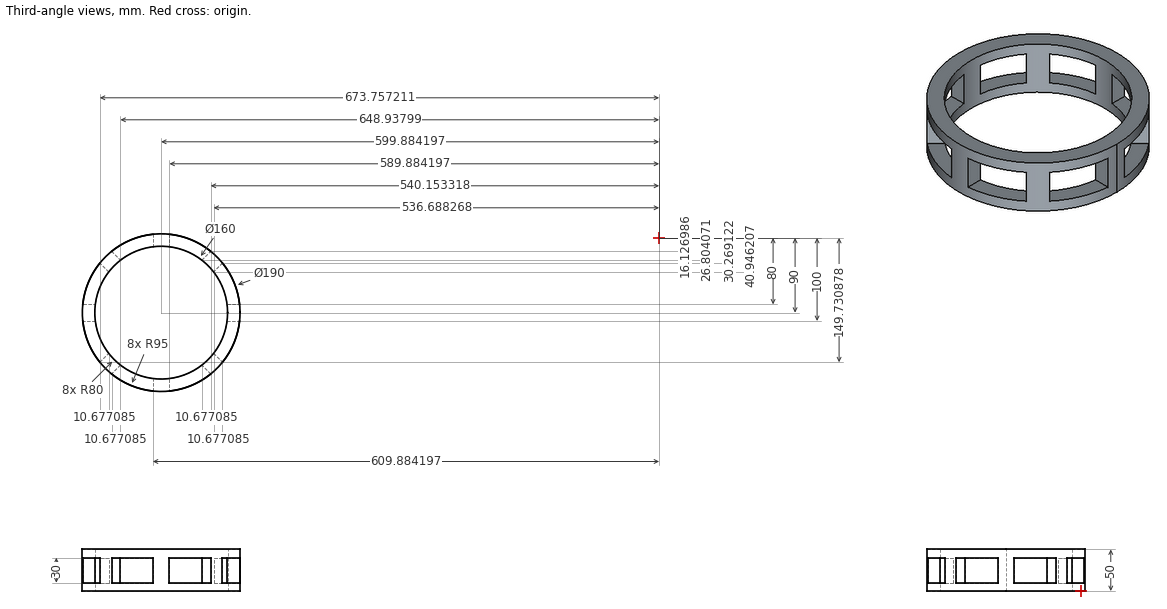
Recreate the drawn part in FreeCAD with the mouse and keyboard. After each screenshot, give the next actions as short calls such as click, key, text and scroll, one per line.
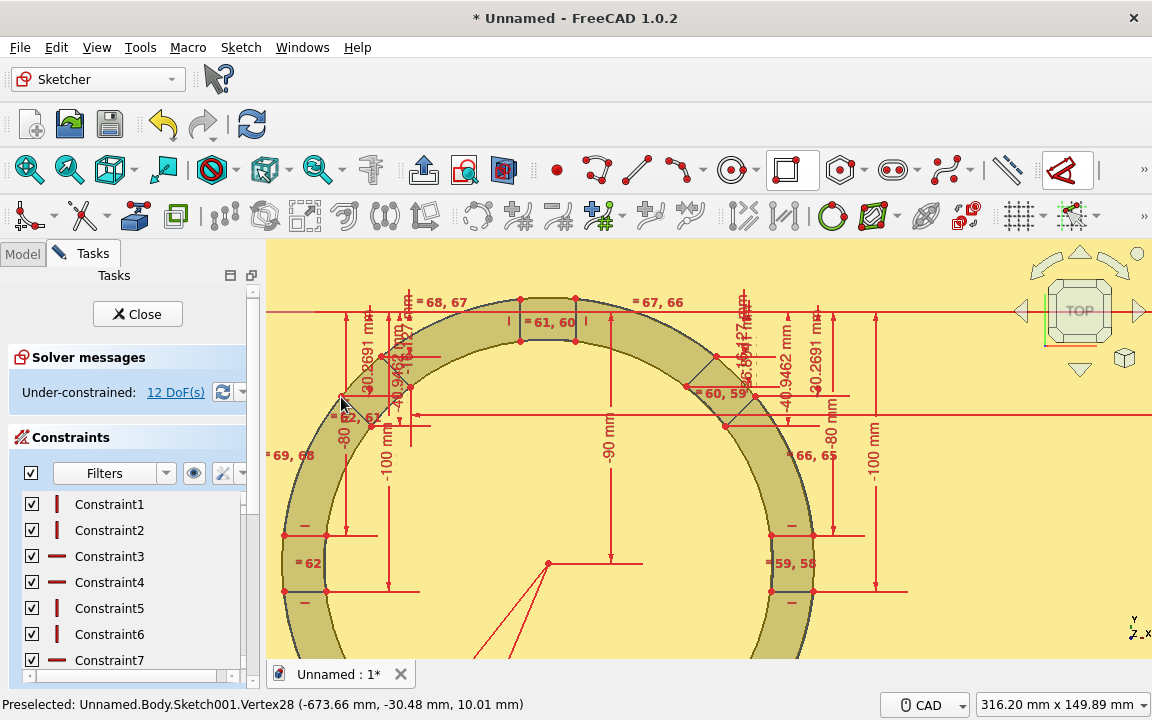
scroll(716, 355, down, 4)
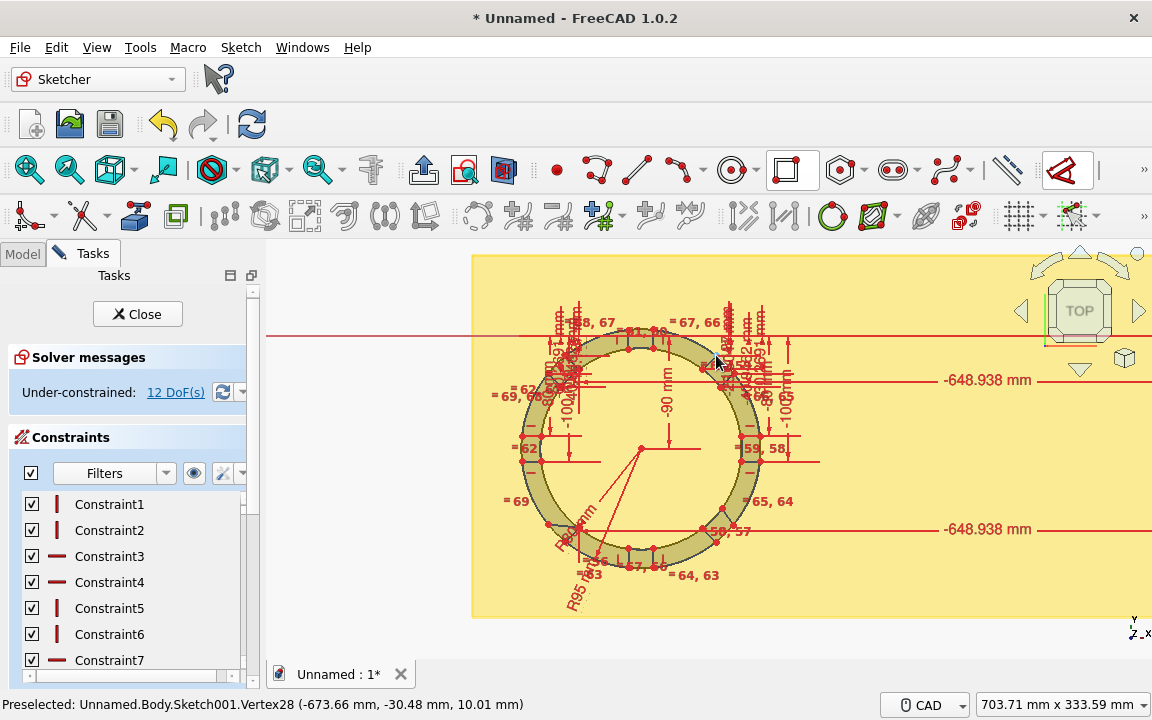
scroll(557, 525, up, 6)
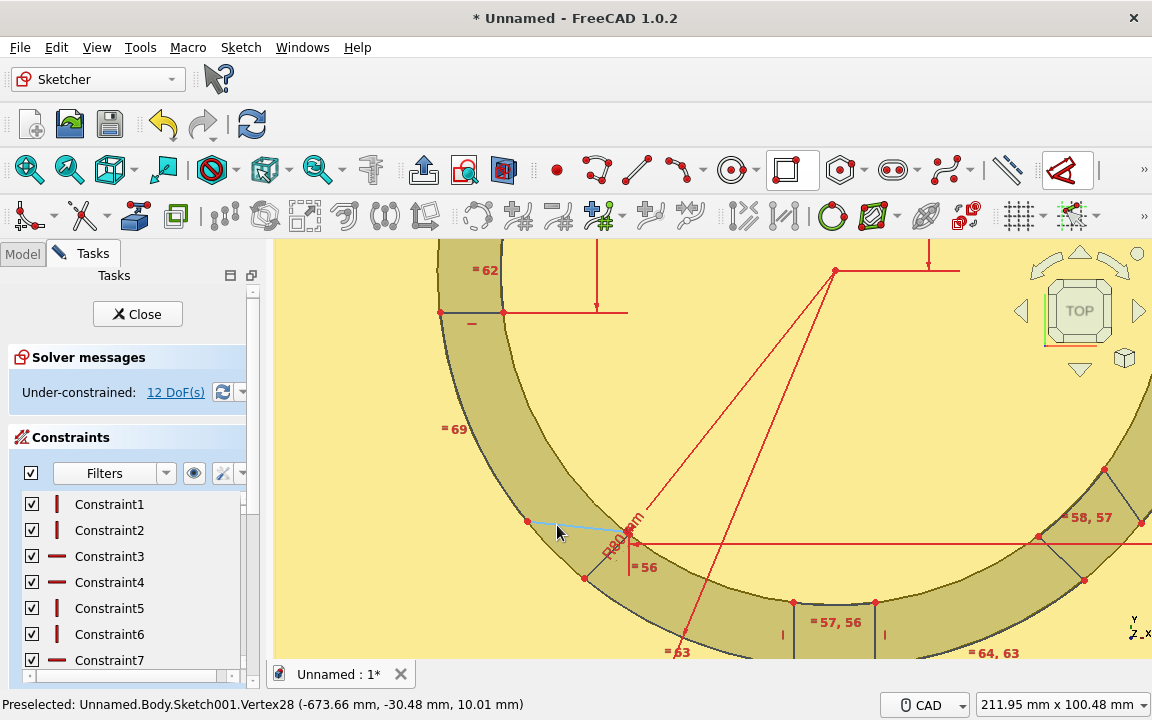
click(557, 525)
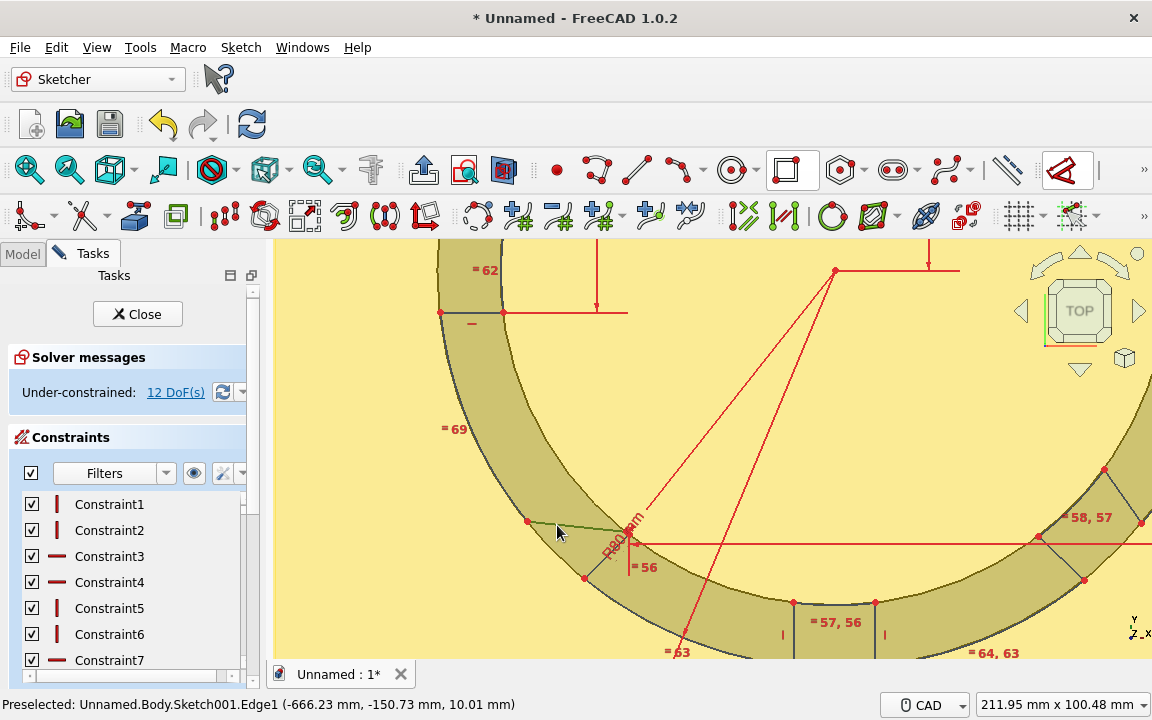
key(l)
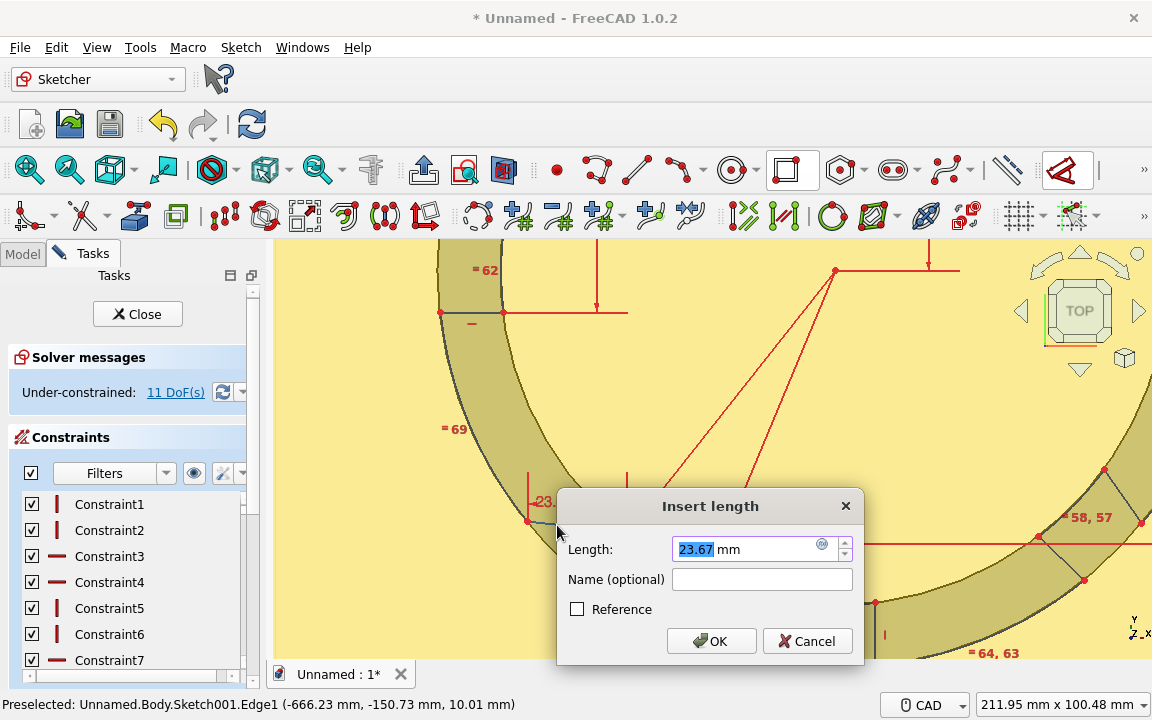
text(10.677085)
key(Return)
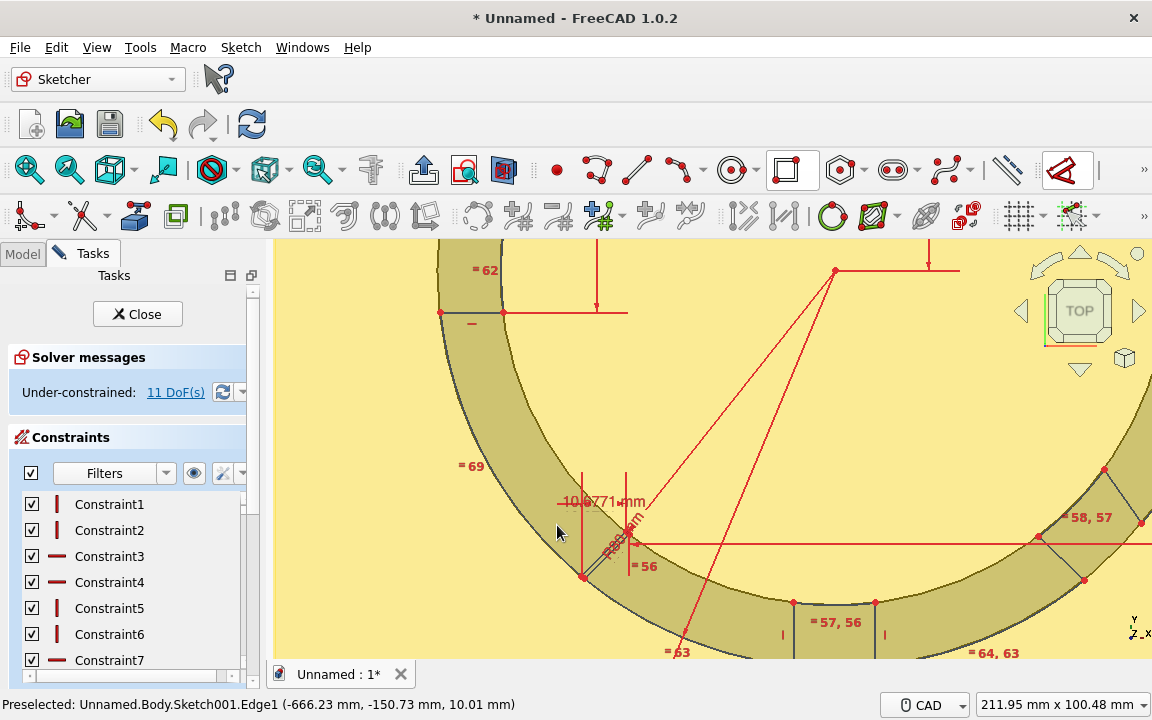
scroll(620, 543, up, 7)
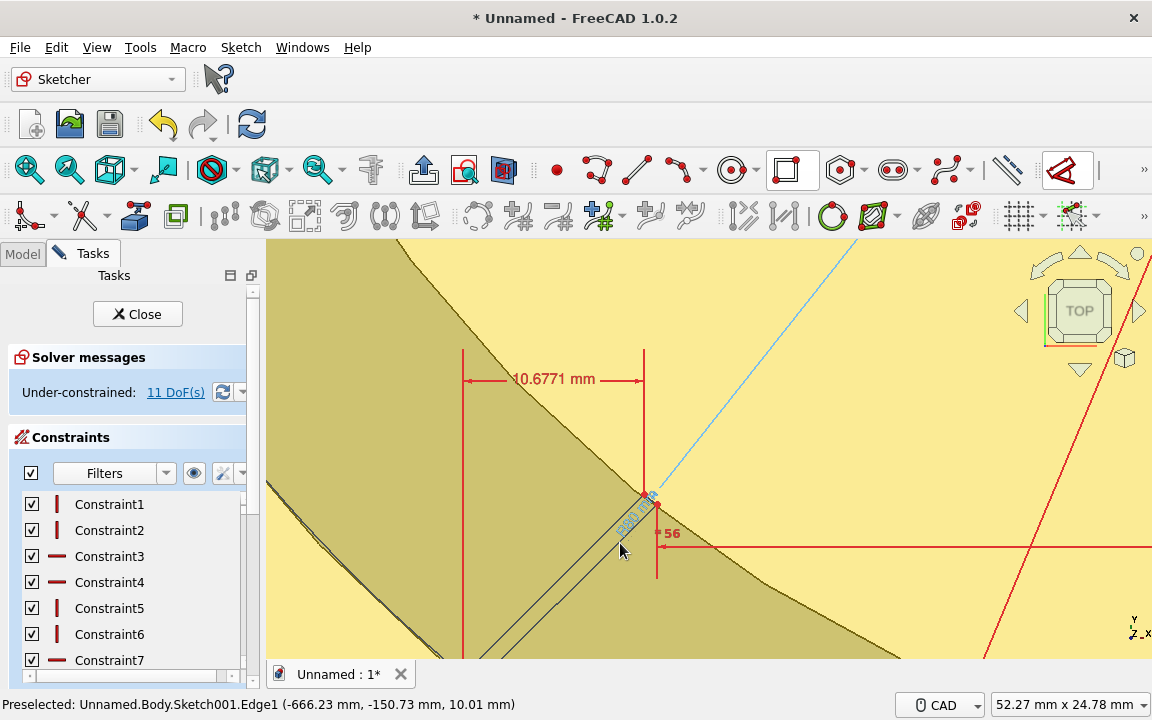
click(621, 541)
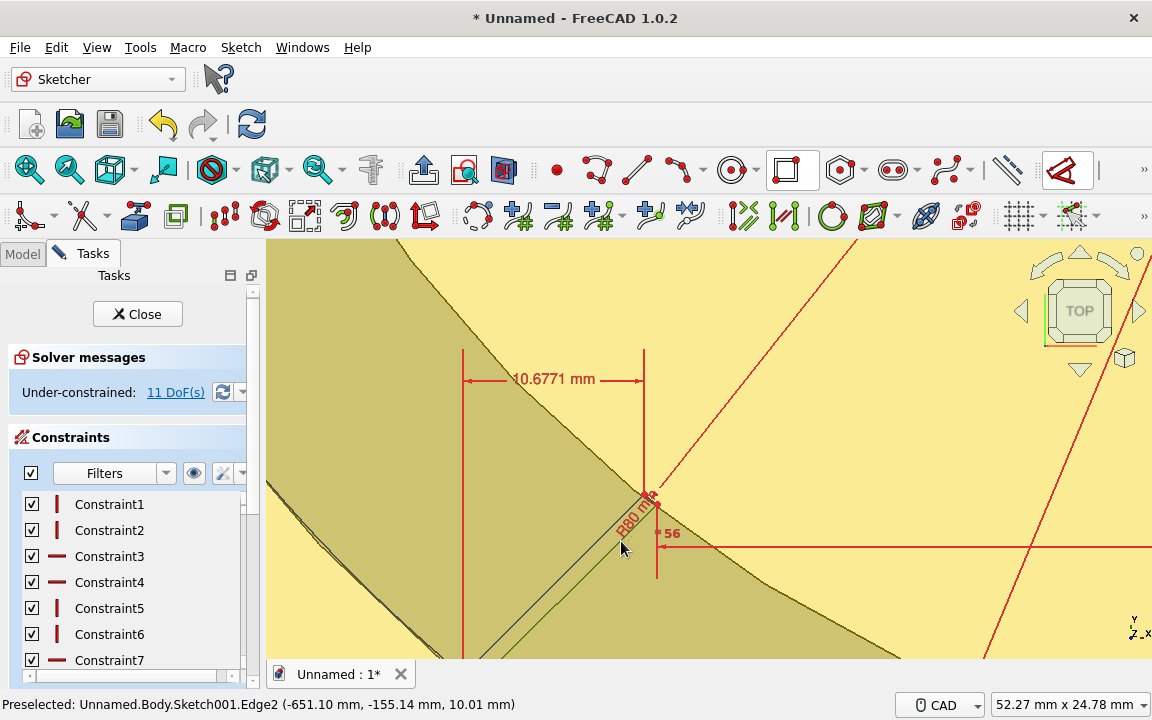
key(l)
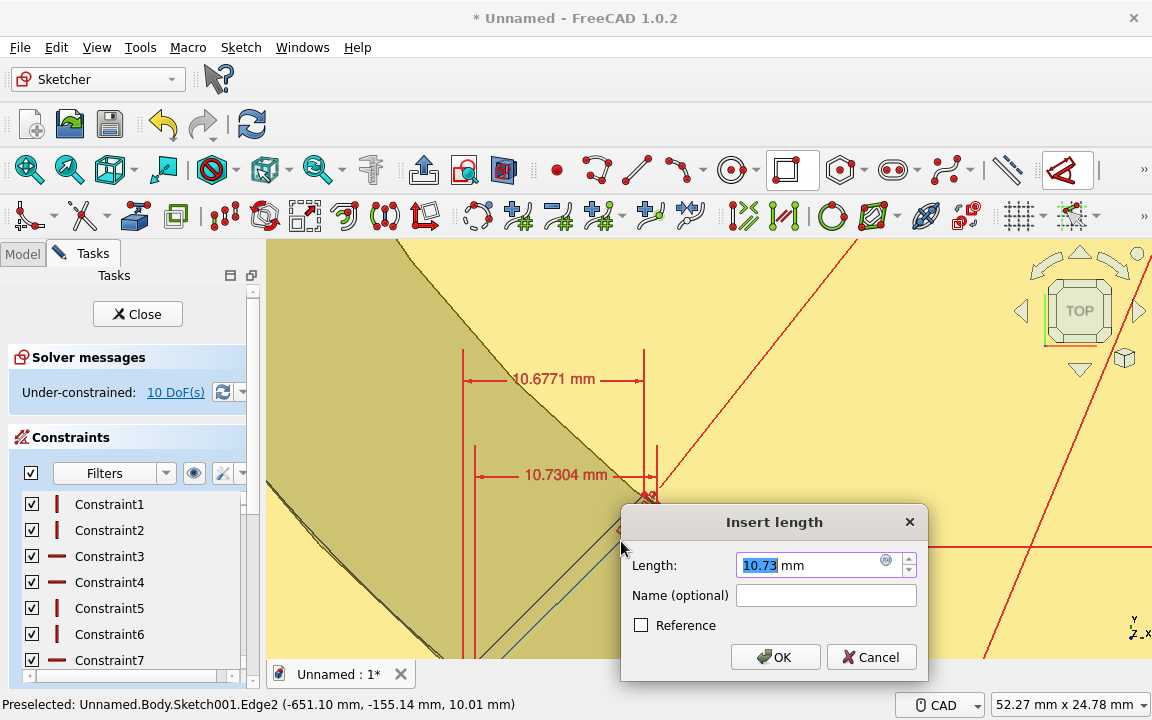
text(10.677085)
key(Return)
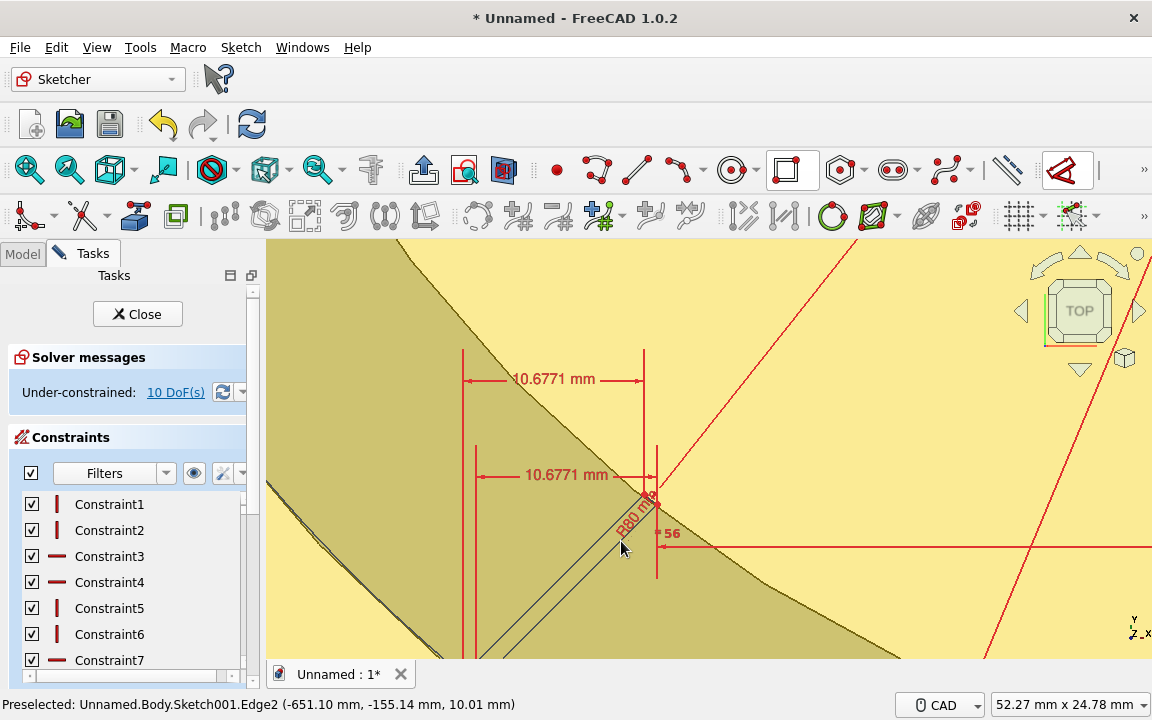
scroll(572, 530, down, 13)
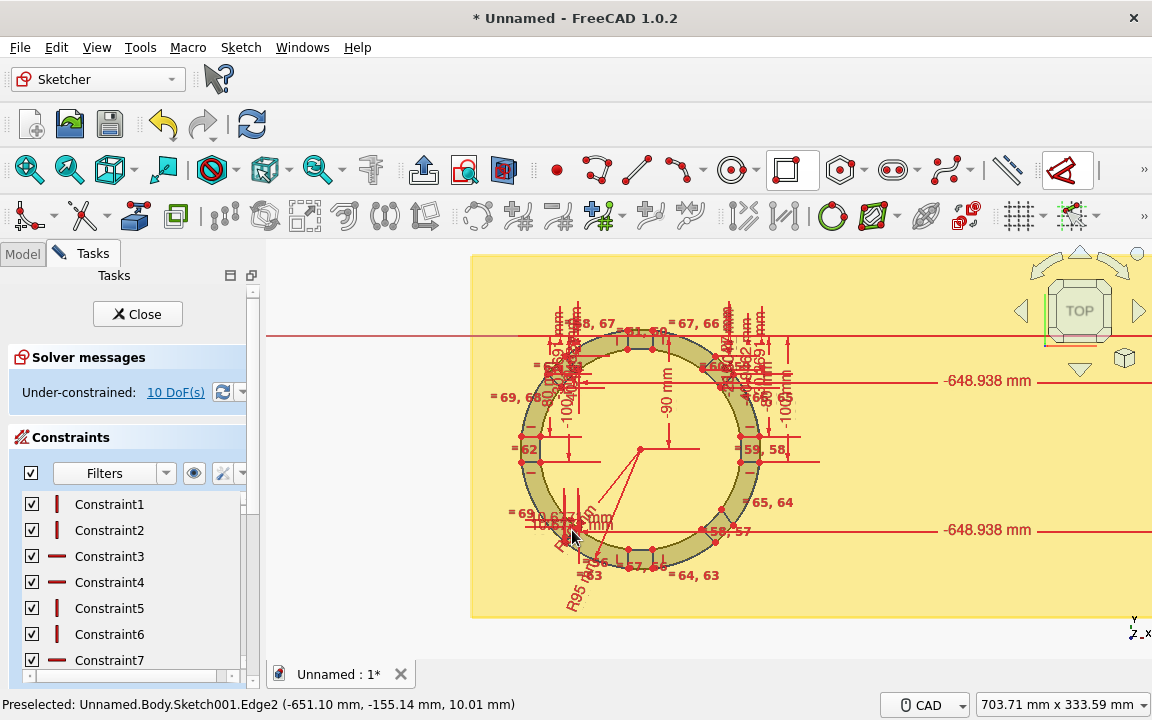
scroll(712, 539, up, 6)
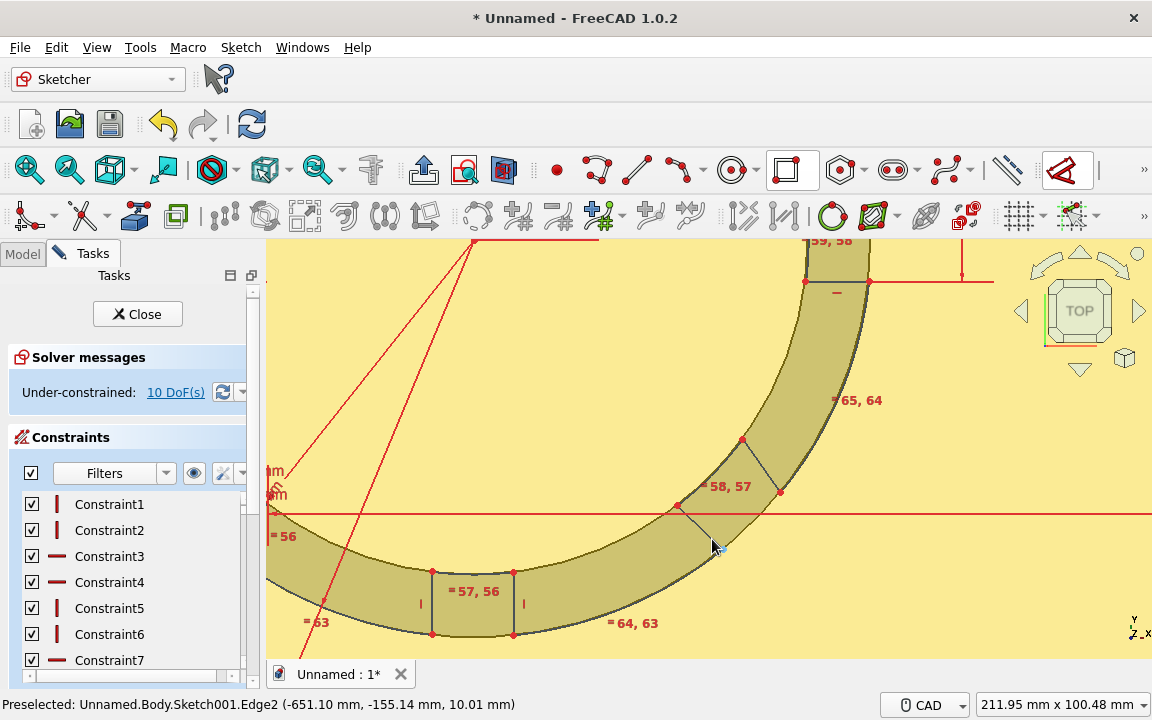
click(709, 536)